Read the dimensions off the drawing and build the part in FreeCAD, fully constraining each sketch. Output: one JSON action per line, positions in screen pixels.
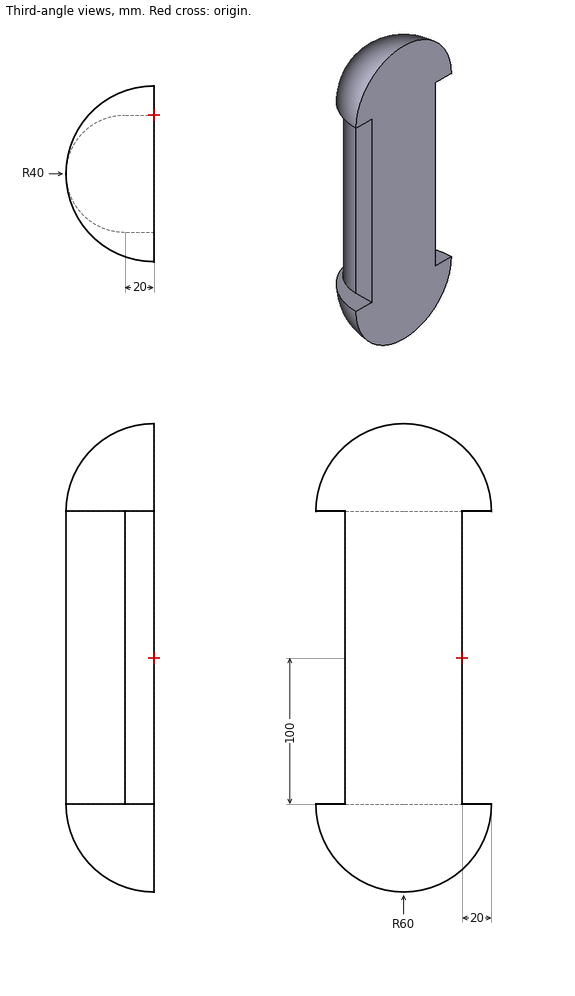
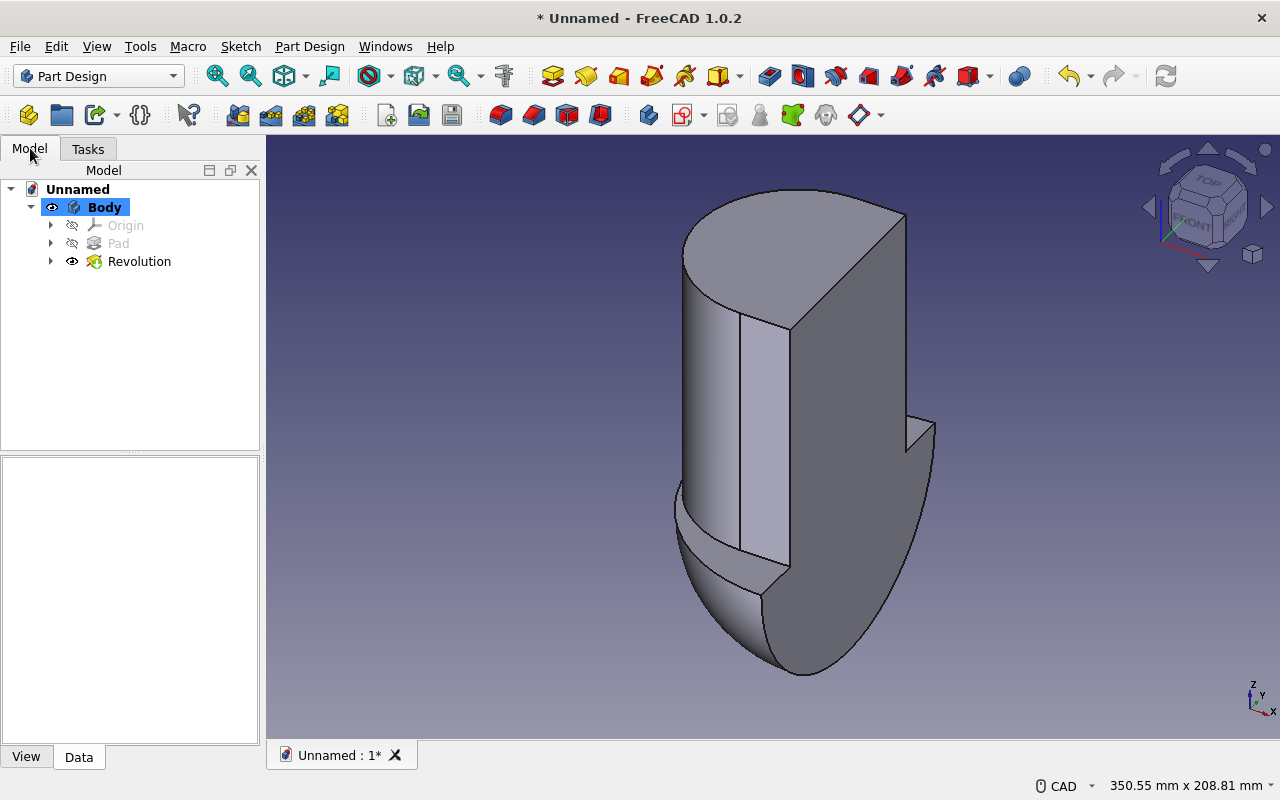
{"action": "left_click", "coordinate": [117, 243]}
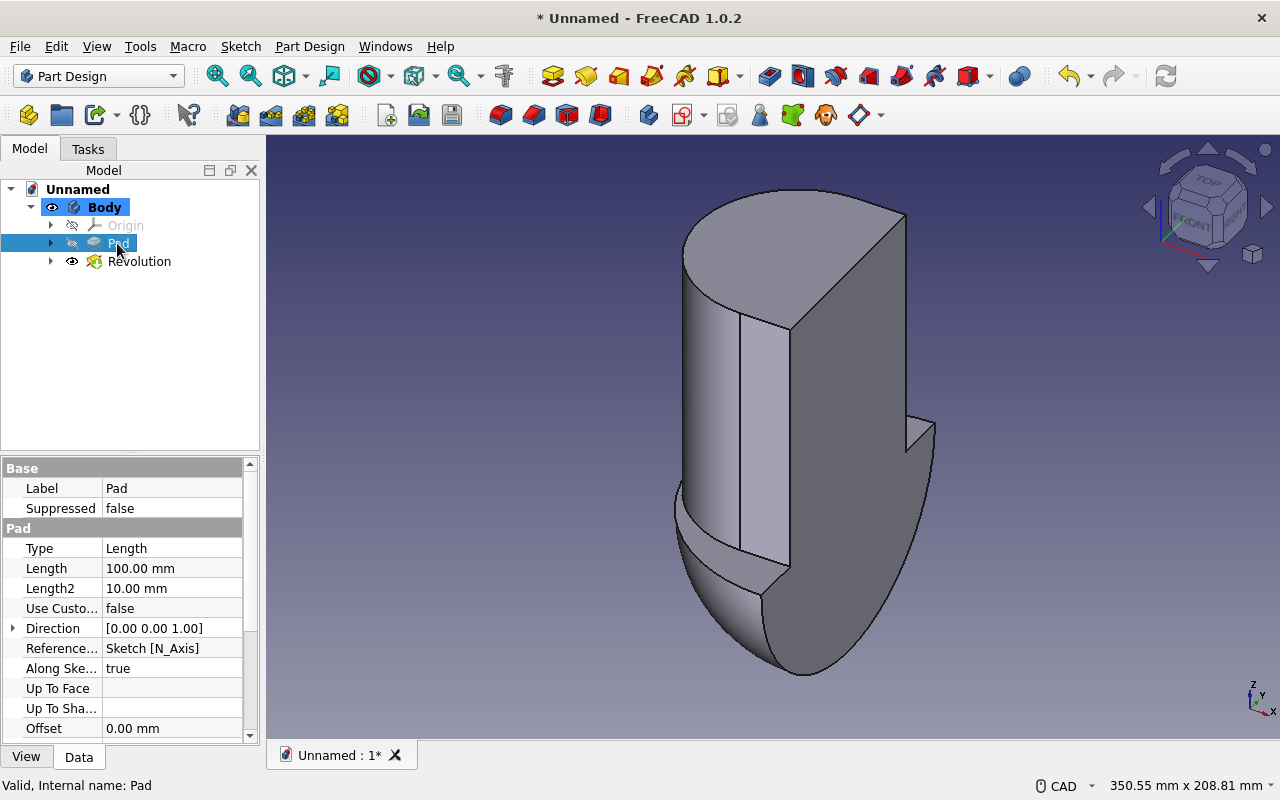
{"action": "left_click", "coordinate": [117, 261], "text": "ctrl"}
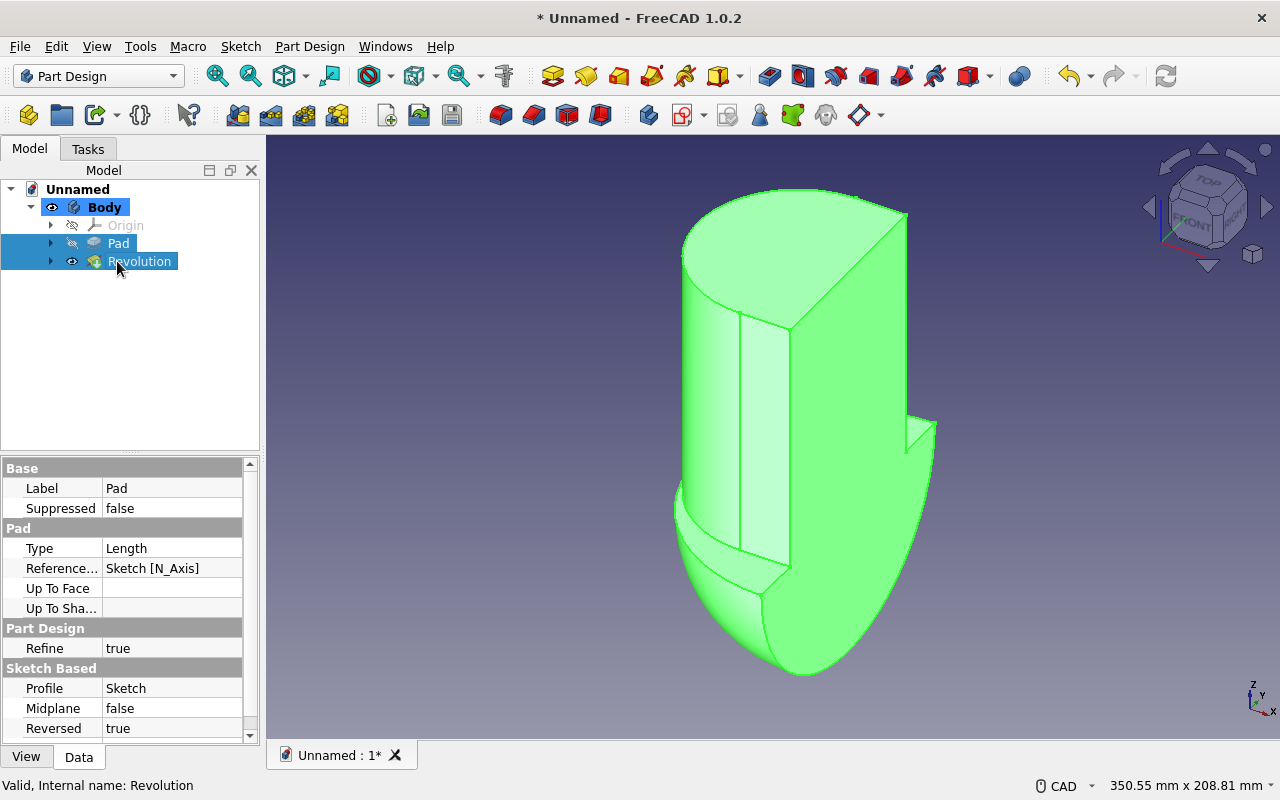
{"action": "left_click", "coordinate": [238, 116]}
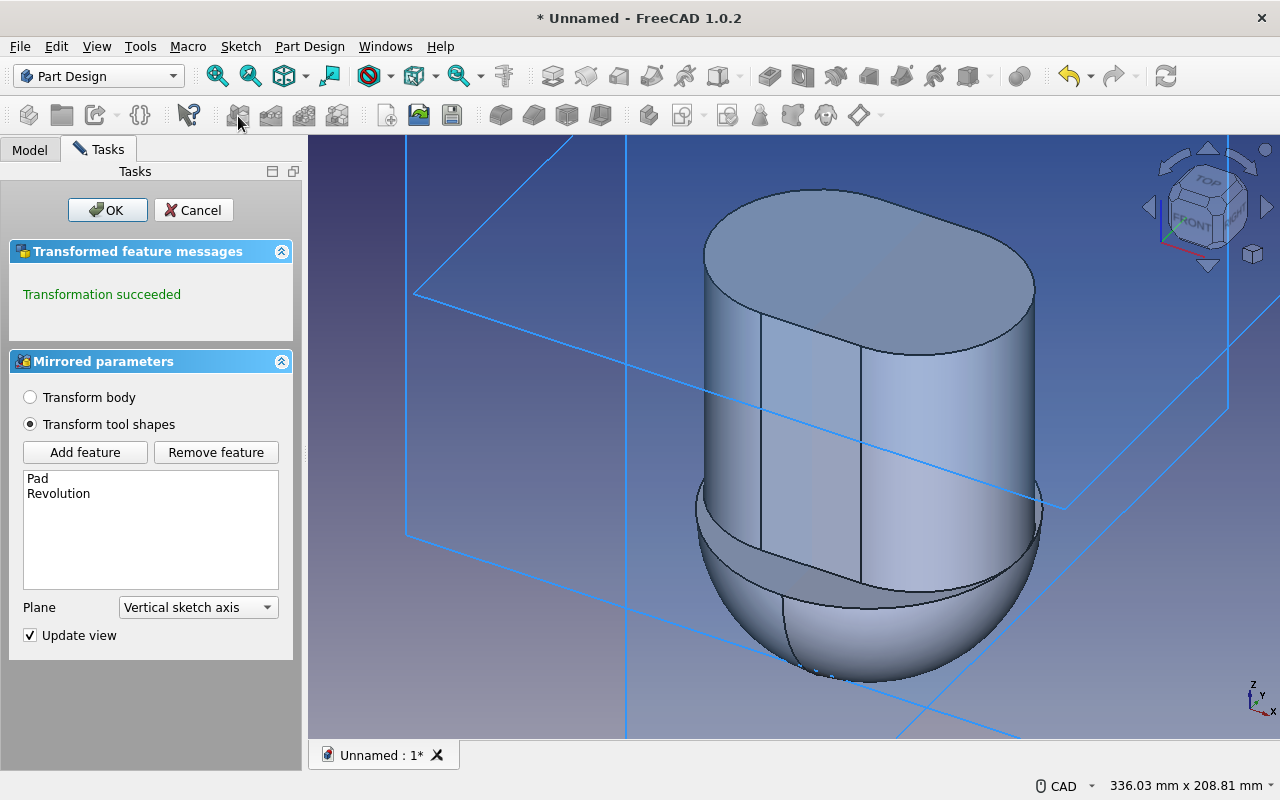
{"action": "left_click", "coordinate": [199, 608]}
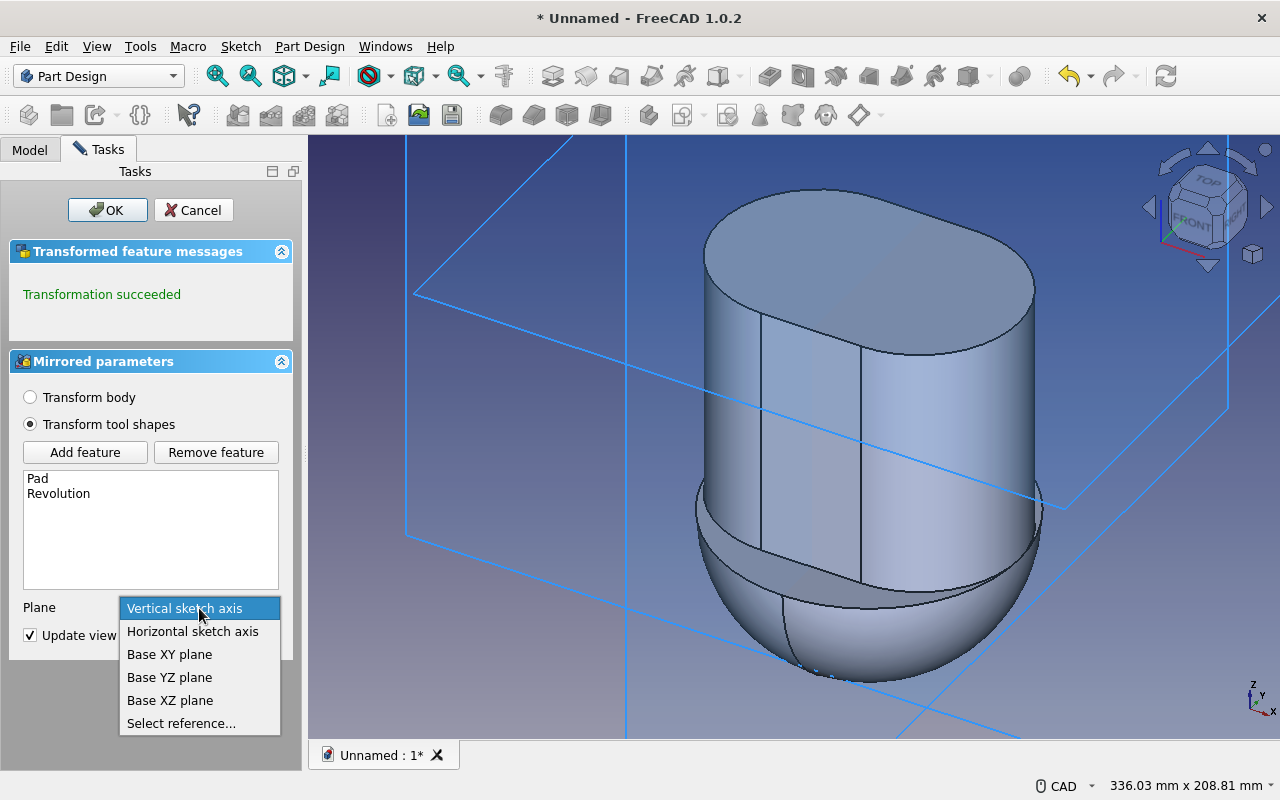
{"action": "left_click", "coordinate": [198, 654]}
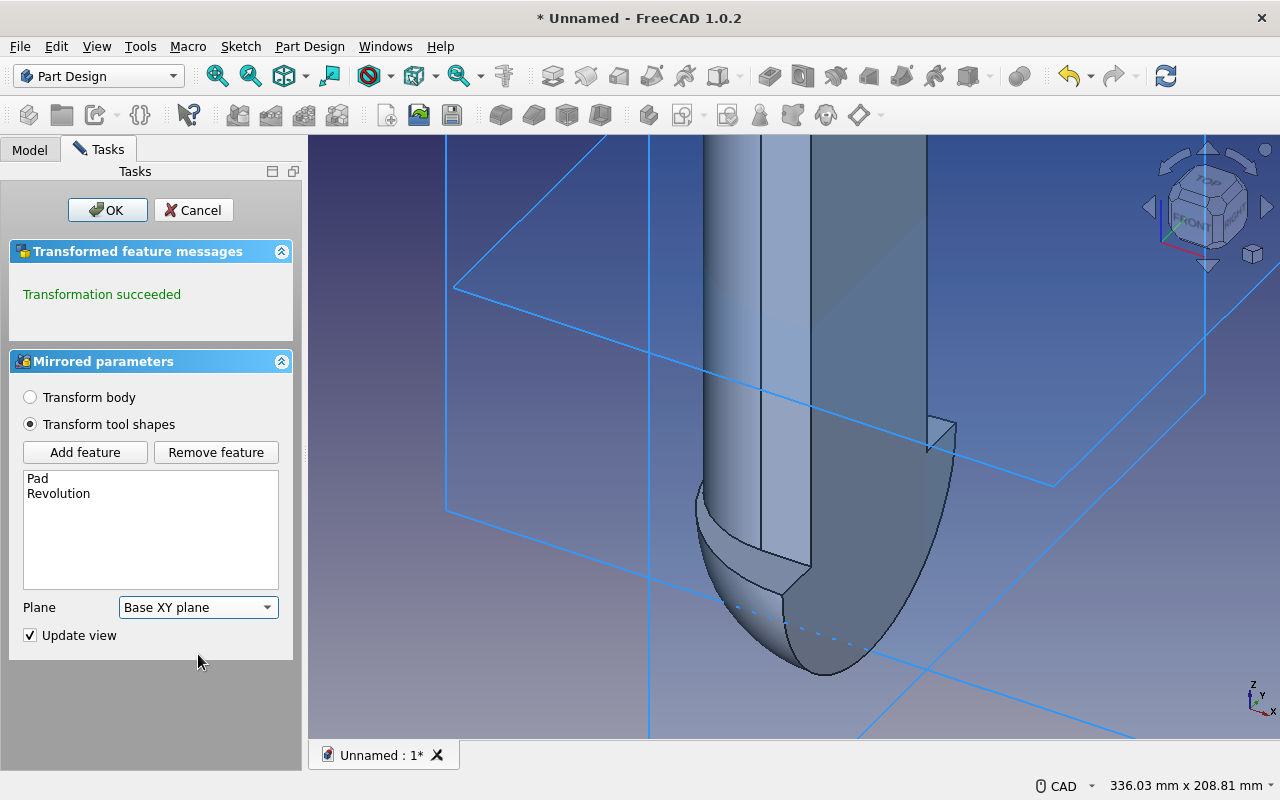
{"action": "left_click", "coordinate": [108, 210]}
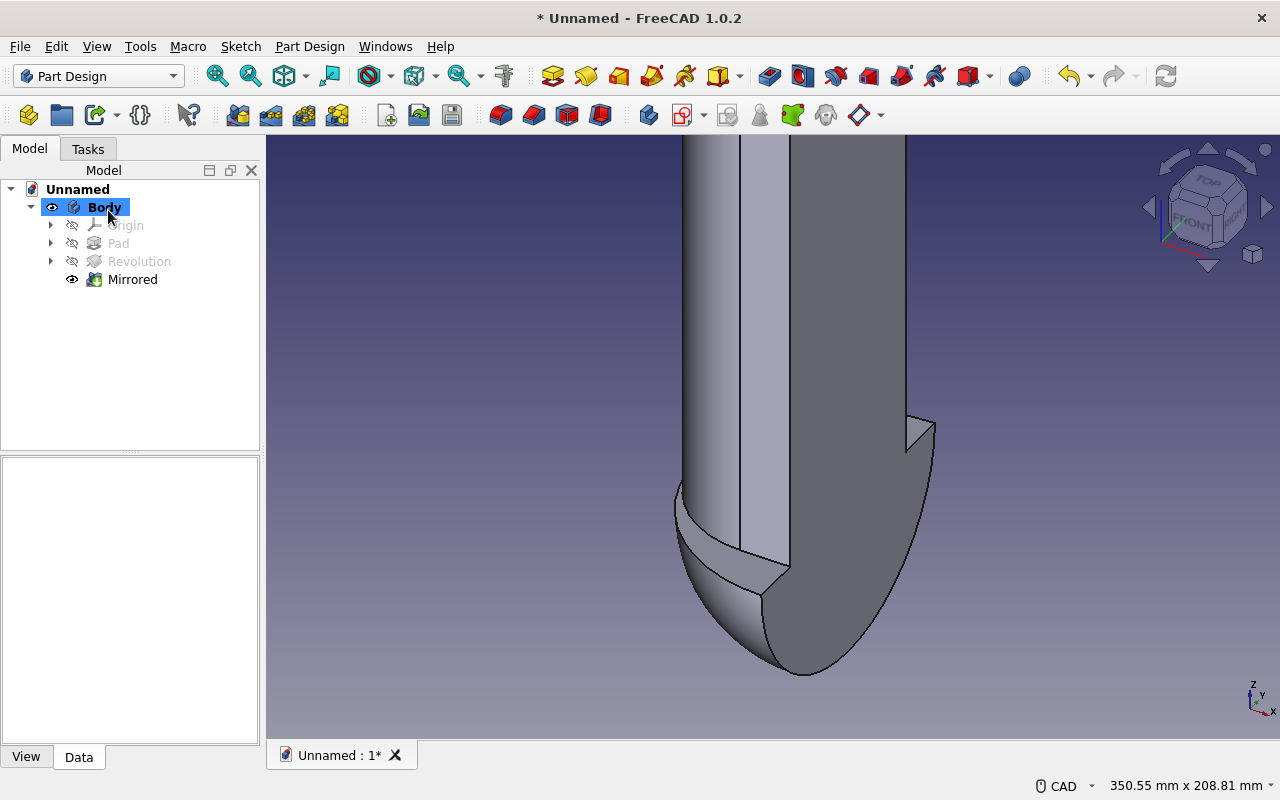
{"action": "key", "text": "0"}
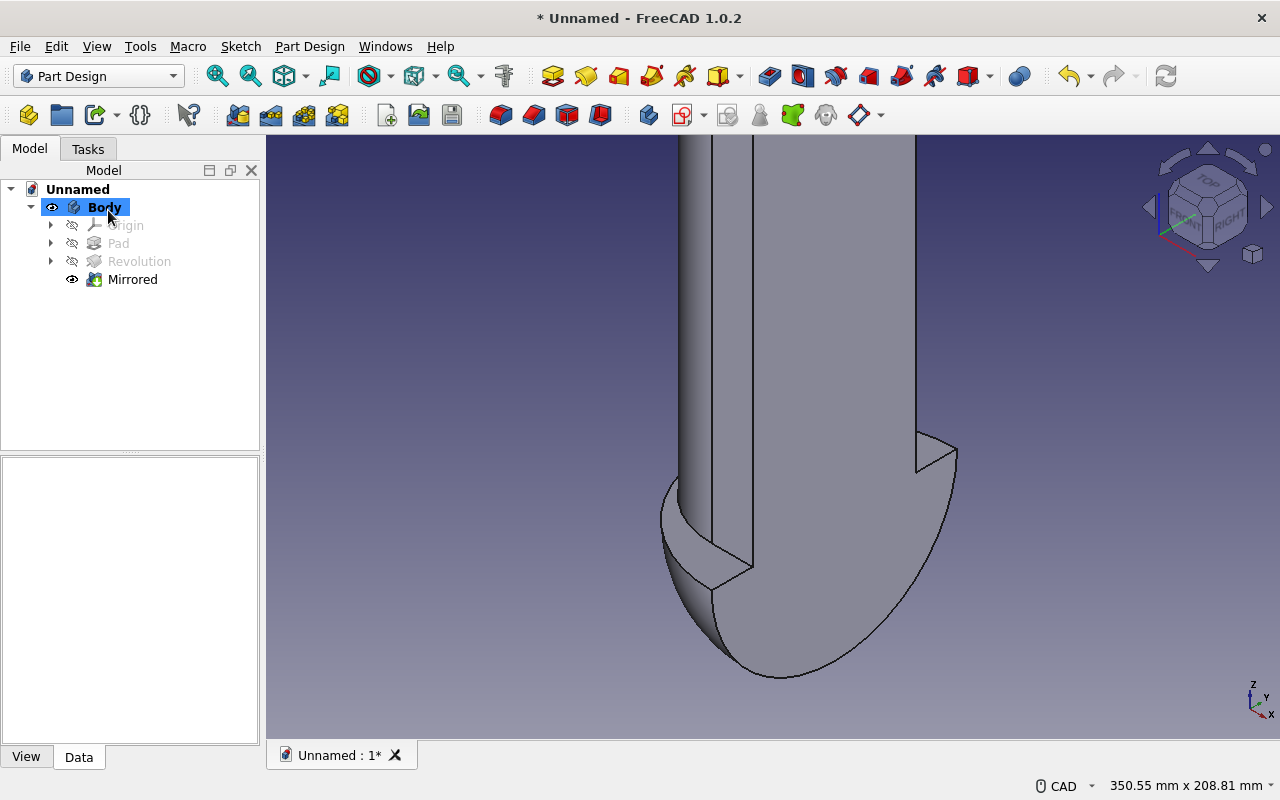
{"action": "key", "text": "v f"}